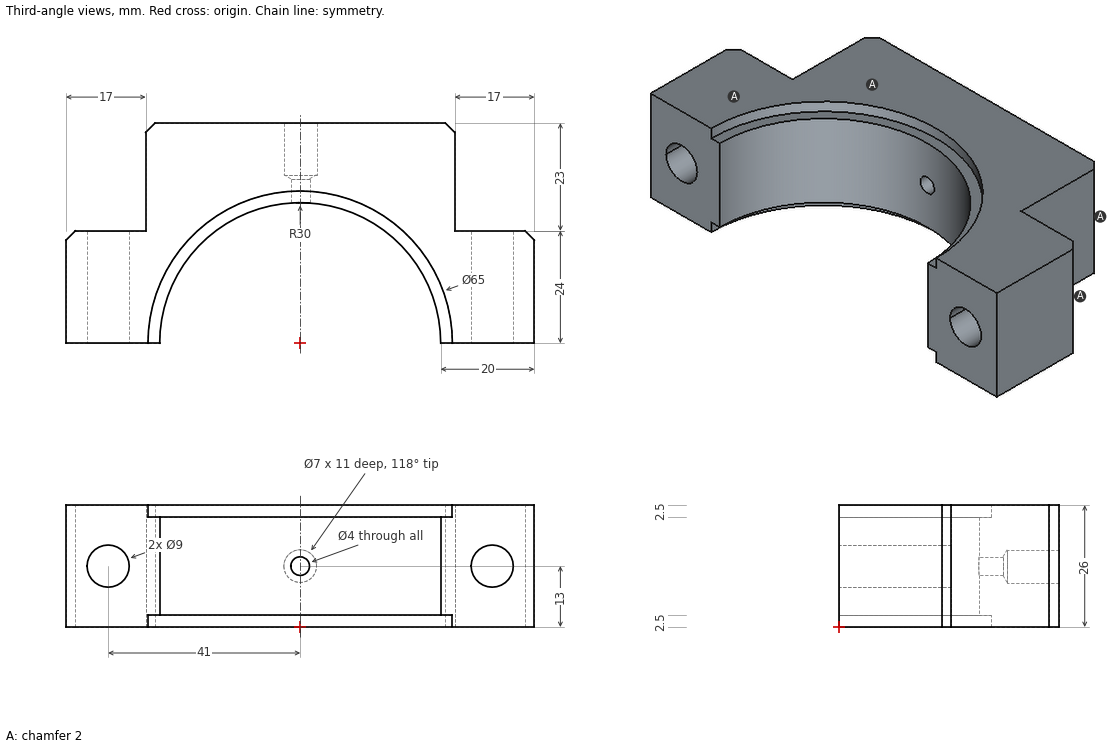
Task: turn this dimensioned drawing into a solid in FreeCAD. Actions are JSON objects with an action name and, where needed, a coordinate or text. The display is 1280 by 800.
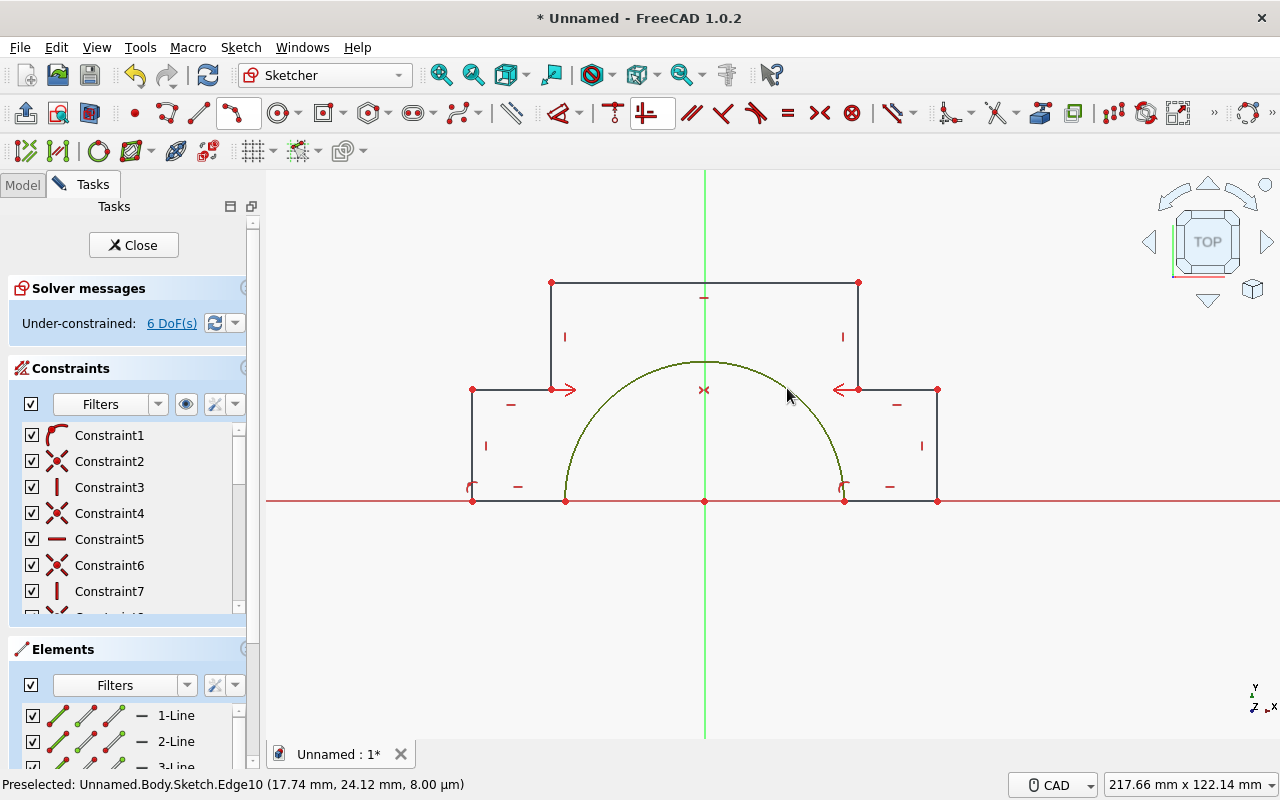
{"action": "key", "text": "k r"}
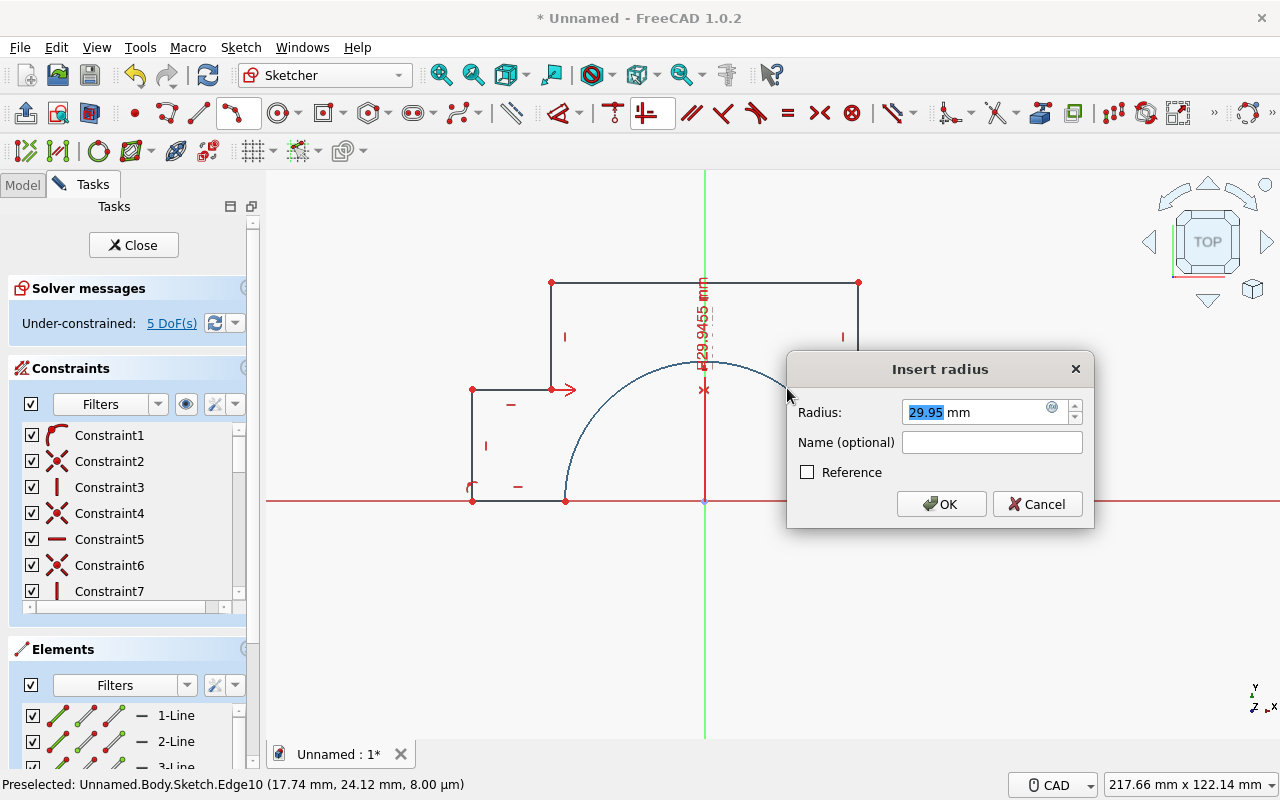
{"action": "type", "text": "30"}
{"action": "key", "text": "Return"}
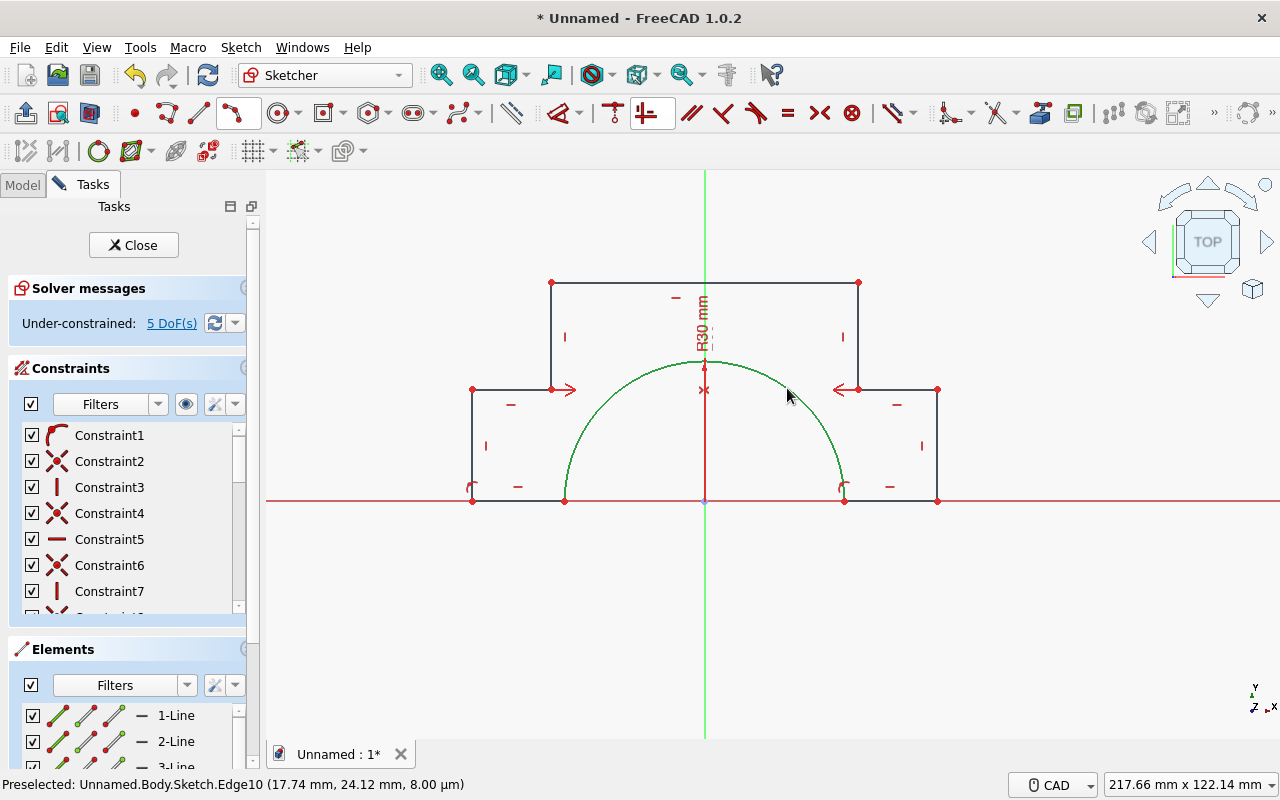
{"action": "left_click", "coordinate": [872, 501]}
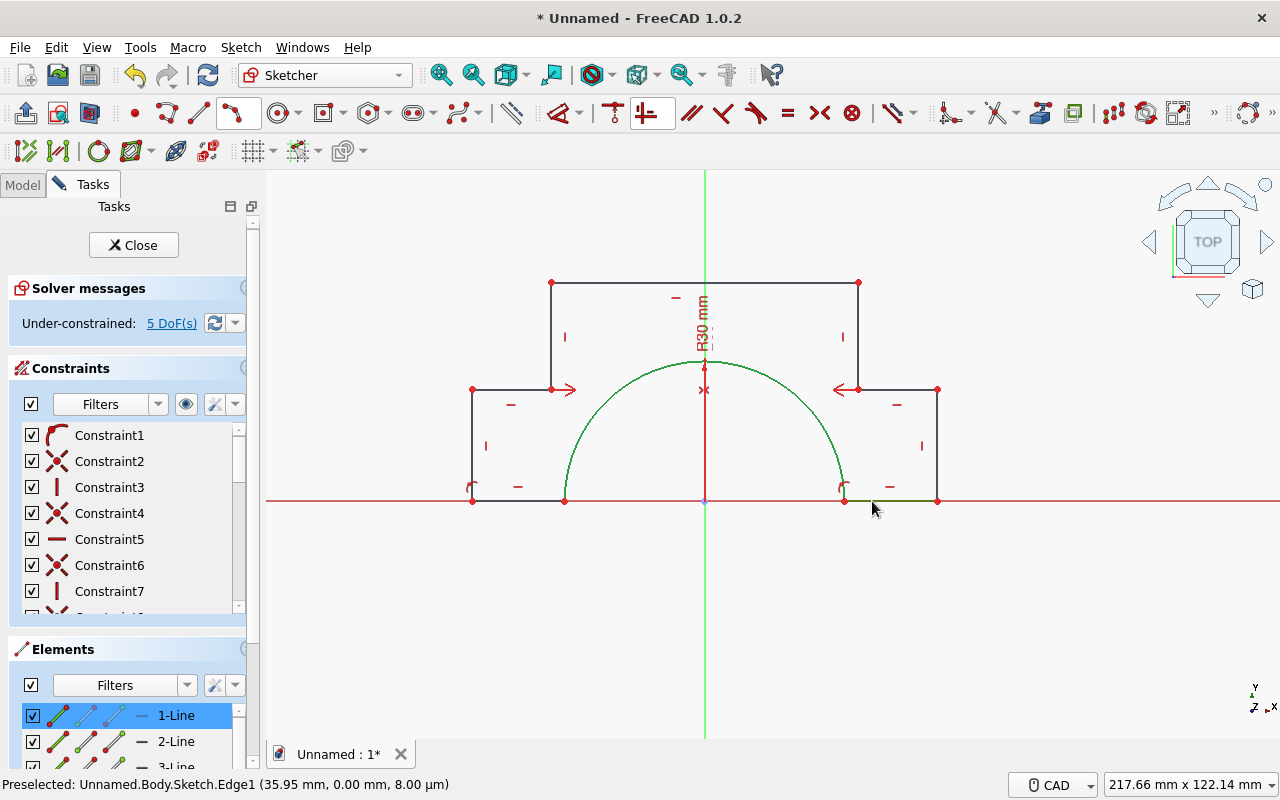
{"action": "key", "text": "l"}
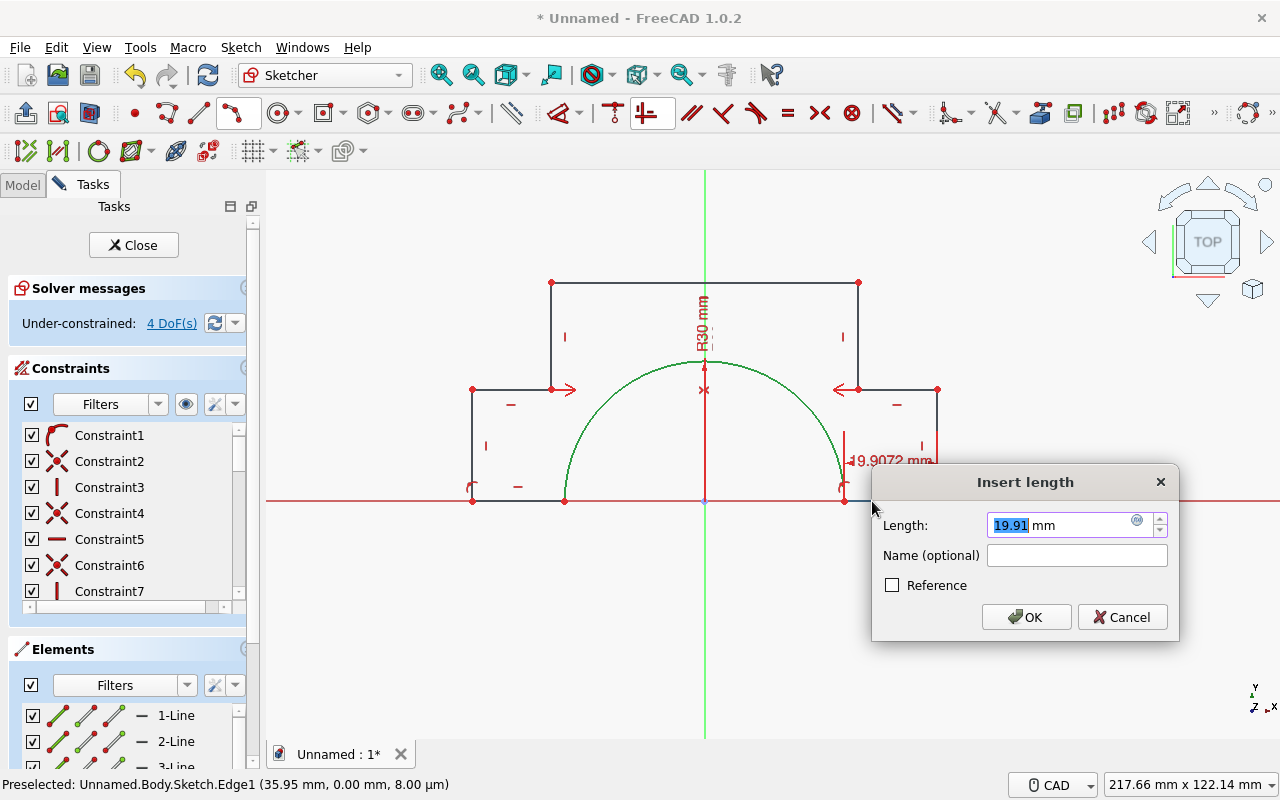
{"action": "type", "text": "20"}
{"action": "key", "text": "Return"}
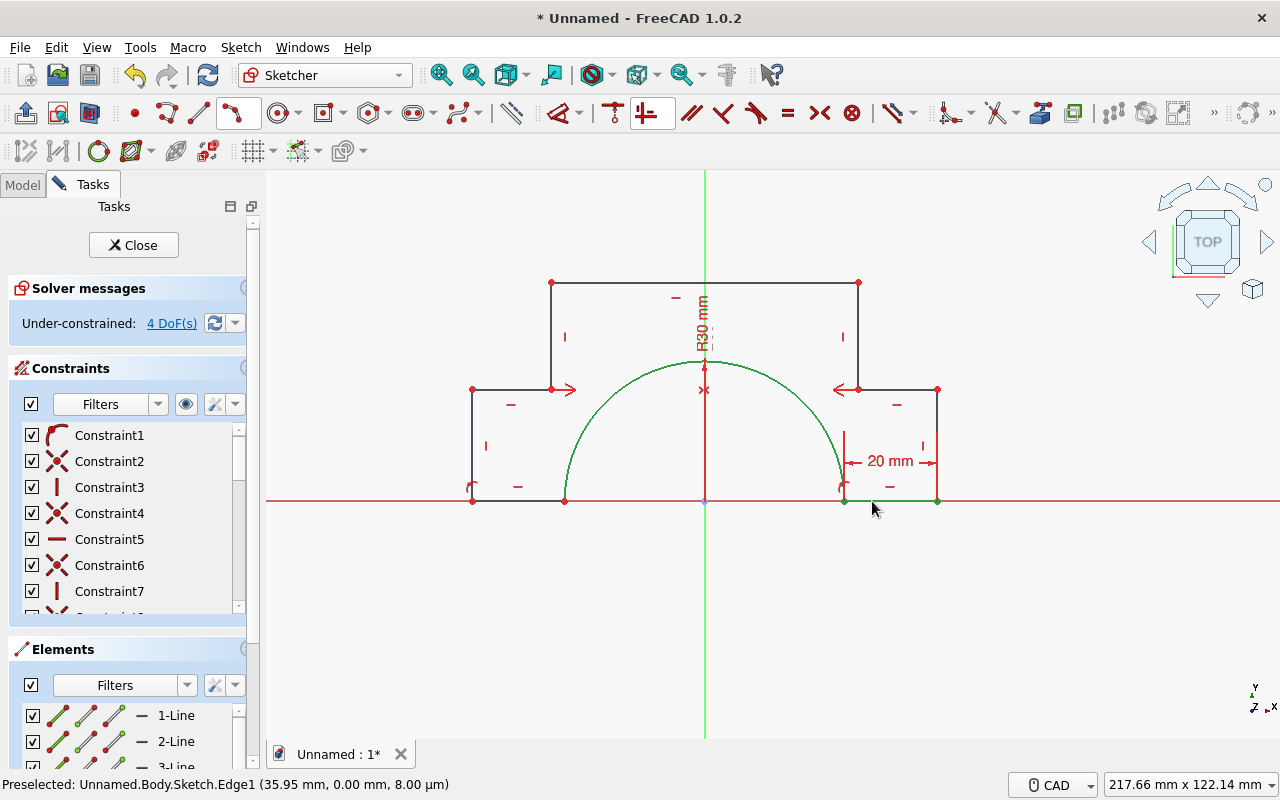
{"action": "left_click", "coordinate": [937, 468]}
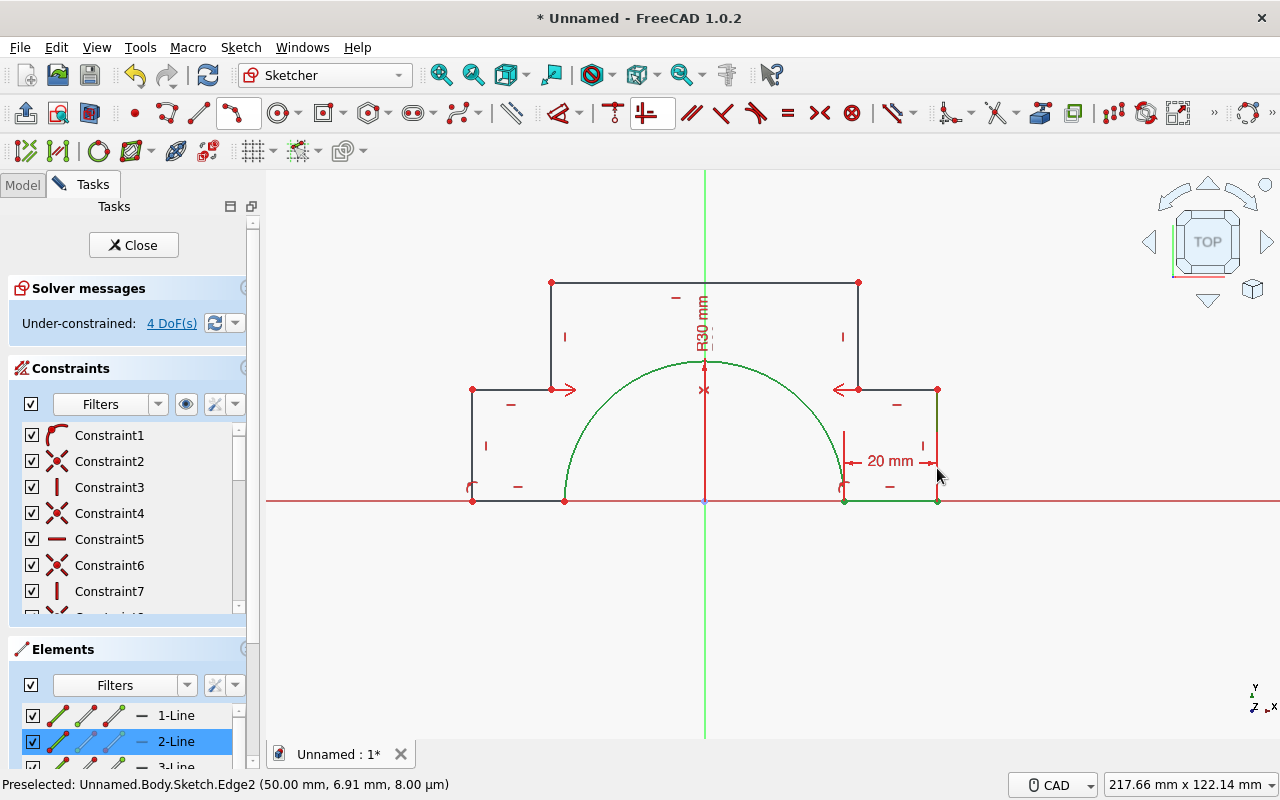
{"action": "key", "text": "i"}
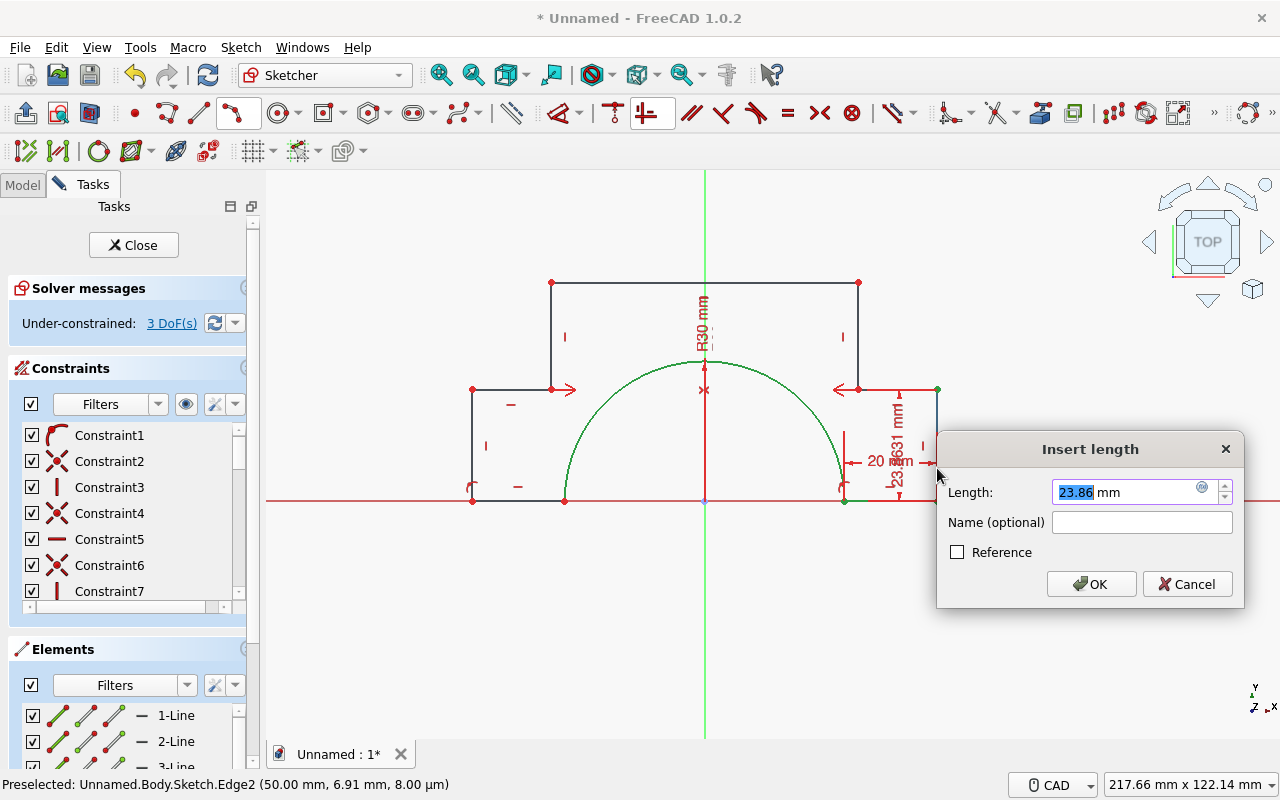
{"action": "type", "text": "24"}
{"action": "key", "text": "Return"}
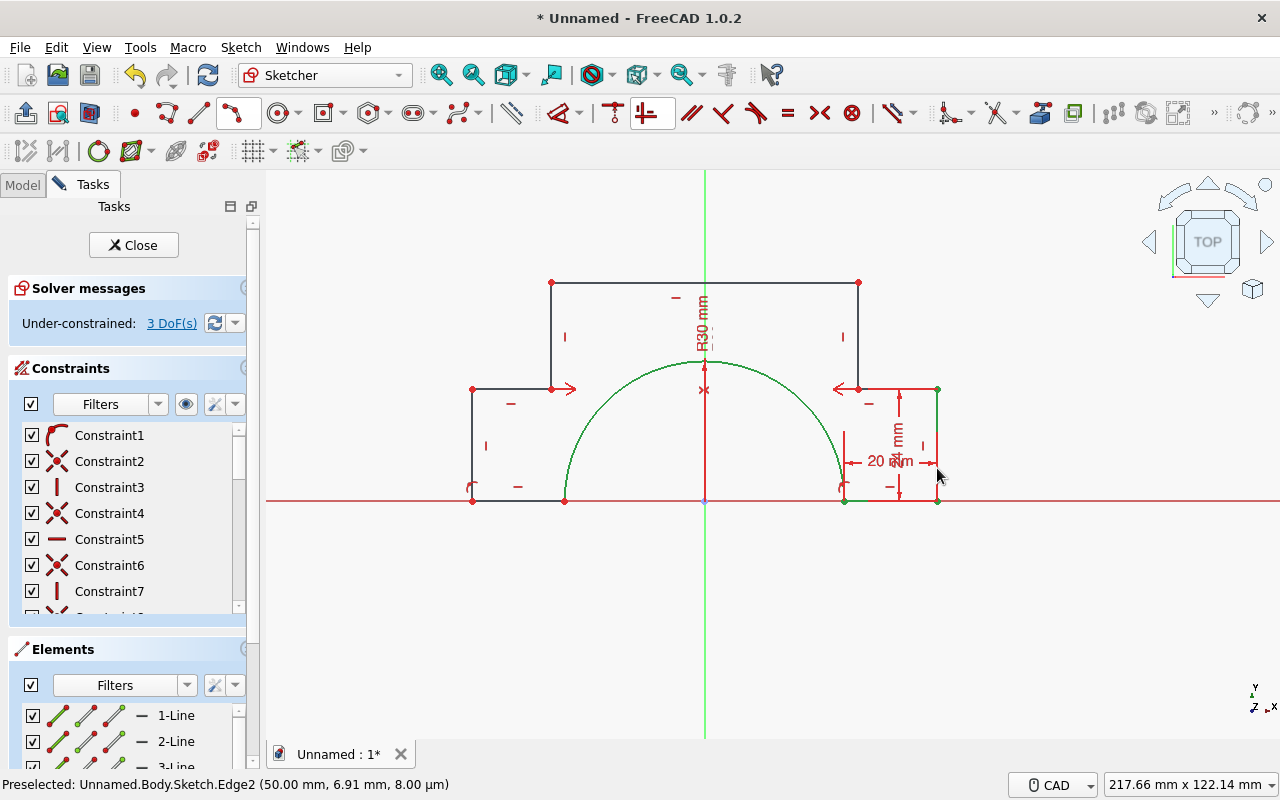
{"action": "left_click", "coordinate": [914, 389]}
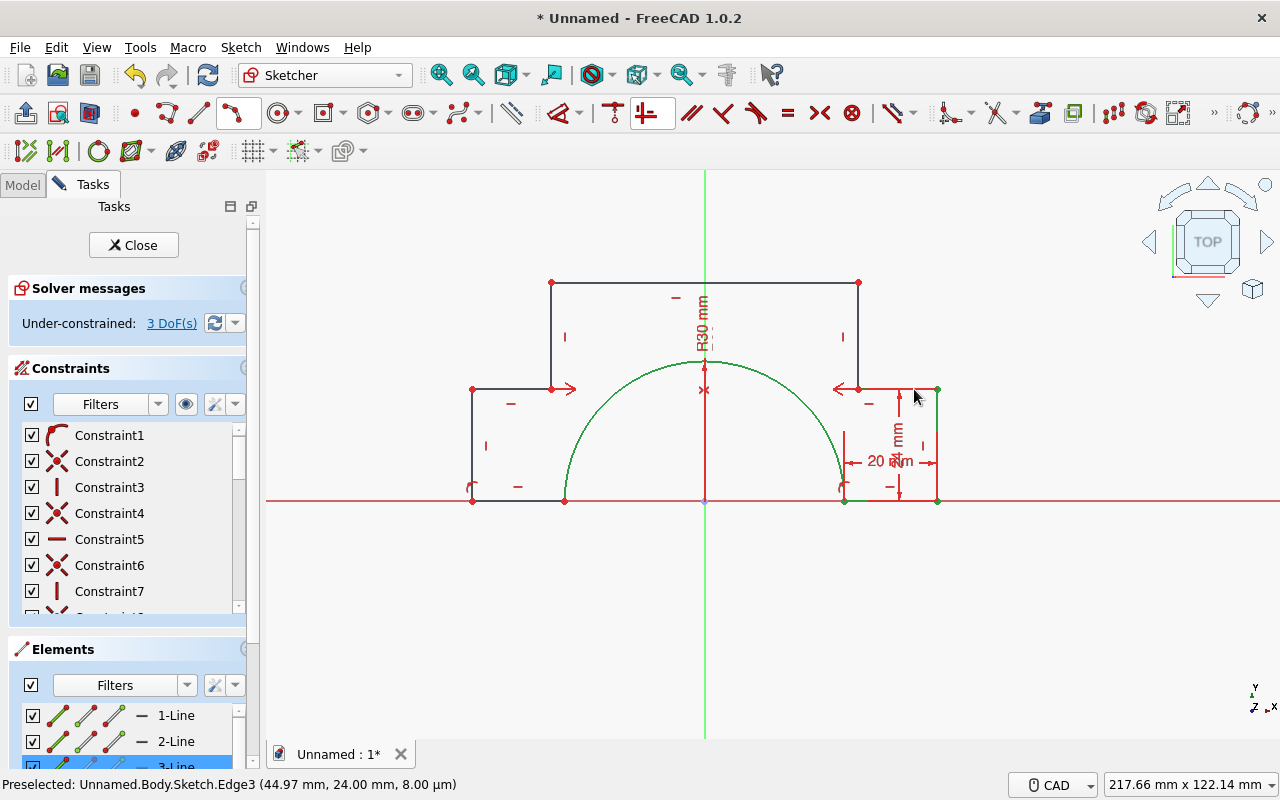
{"action": "left_click", "coordinate": [582, 114]}